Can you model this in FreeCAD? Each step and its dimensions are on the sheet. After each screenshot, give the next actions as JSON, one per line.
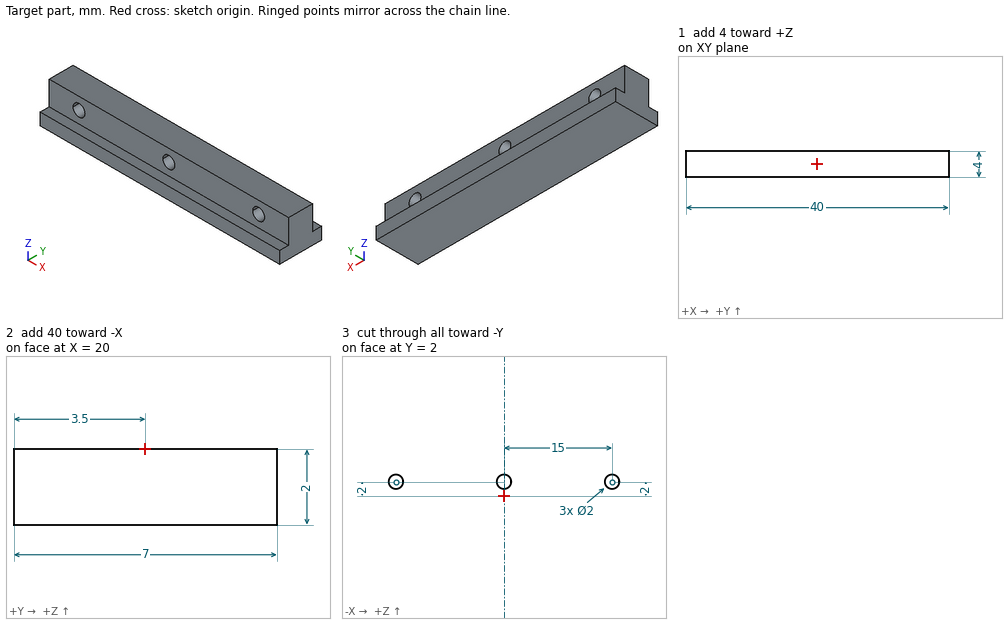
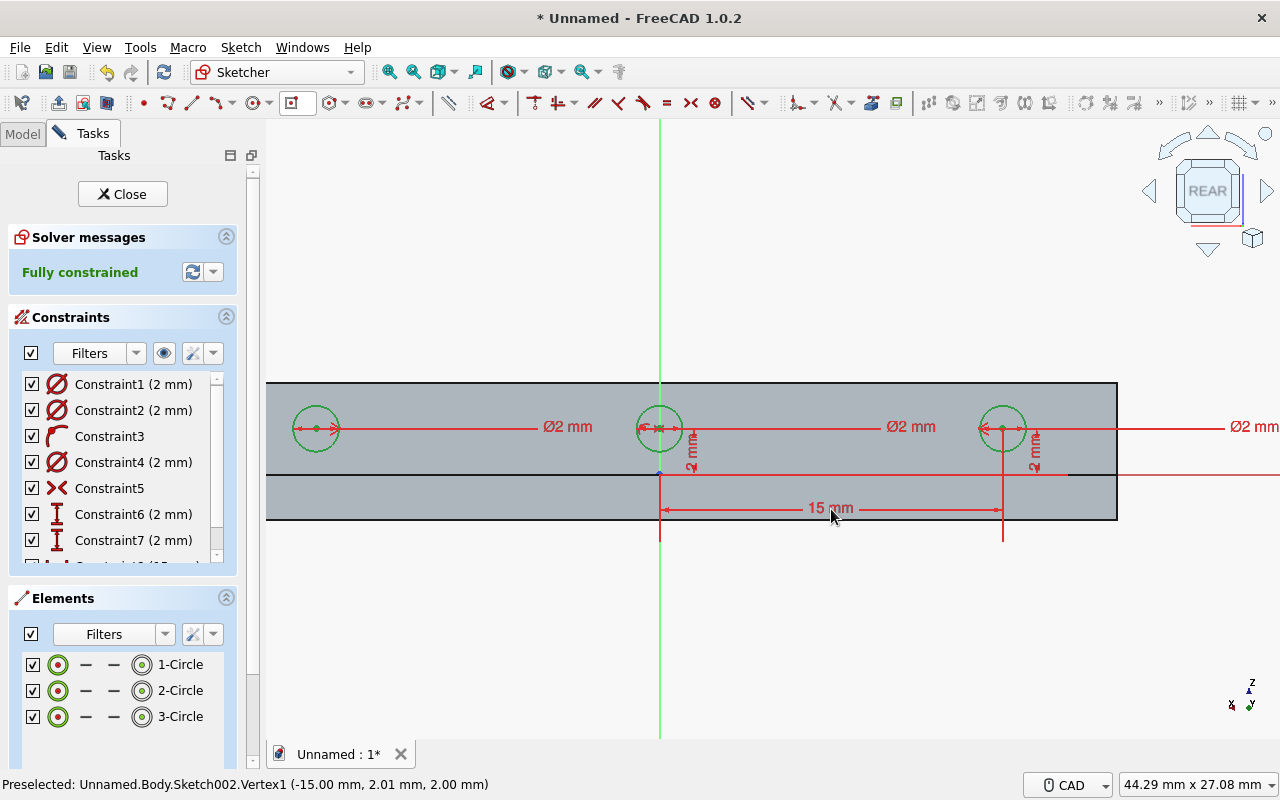
{"action": "left_click", "coordinate": [123, 194]}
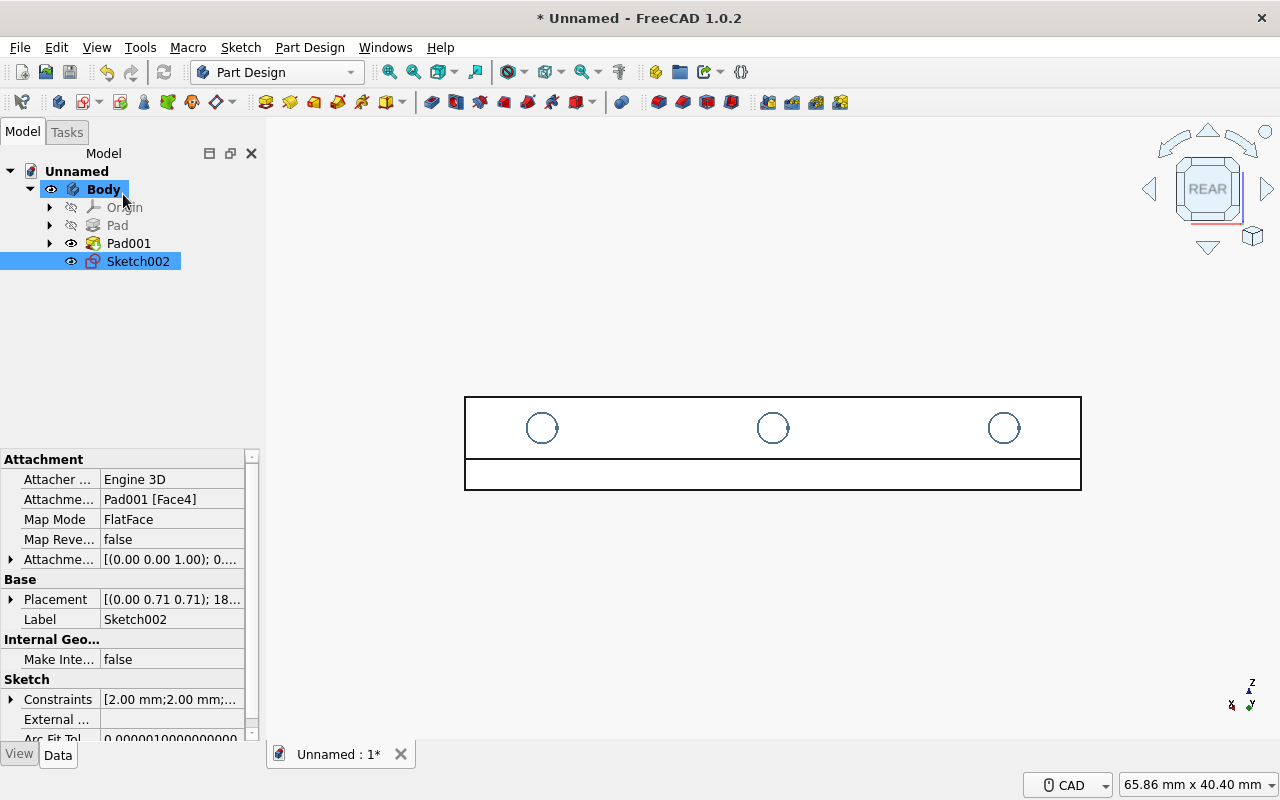
{"action": "left_click", "coordinate": [432, 102]}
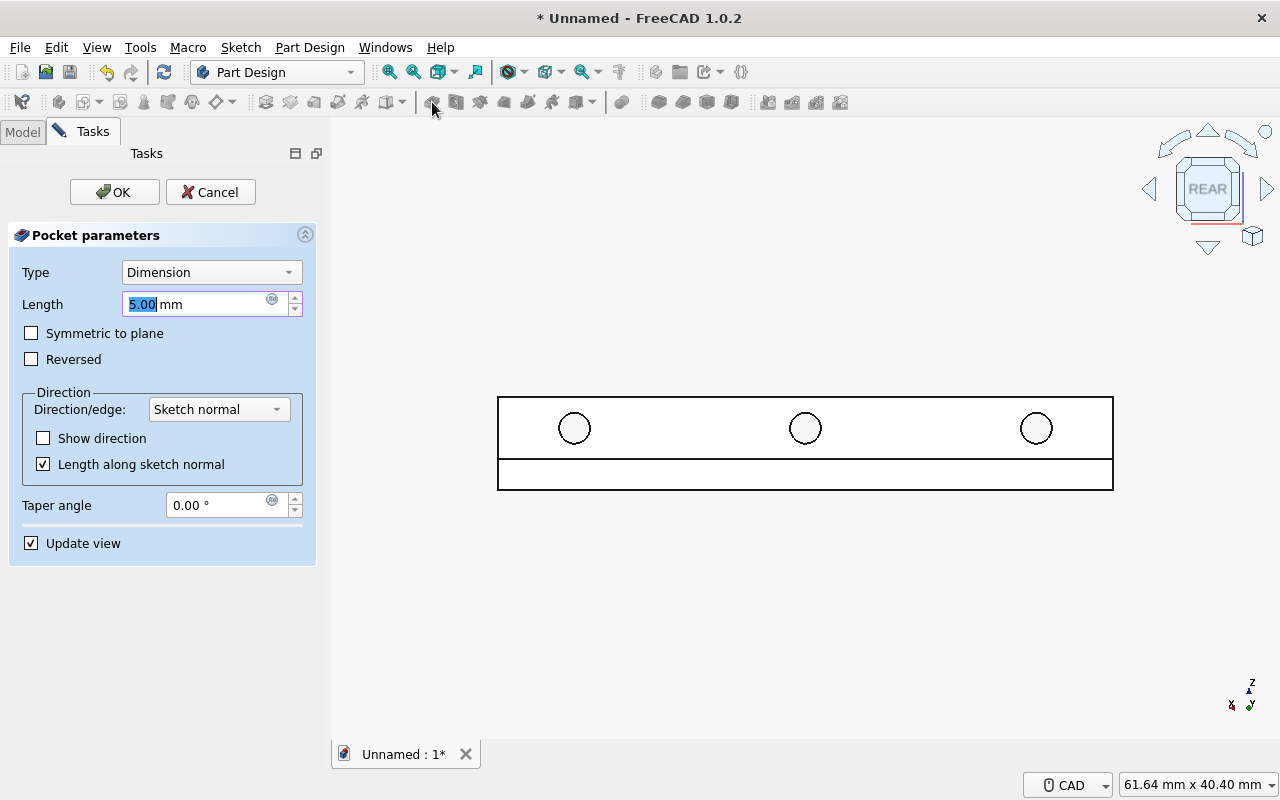
{"action": "left_click", "coordinate": [212, 272]}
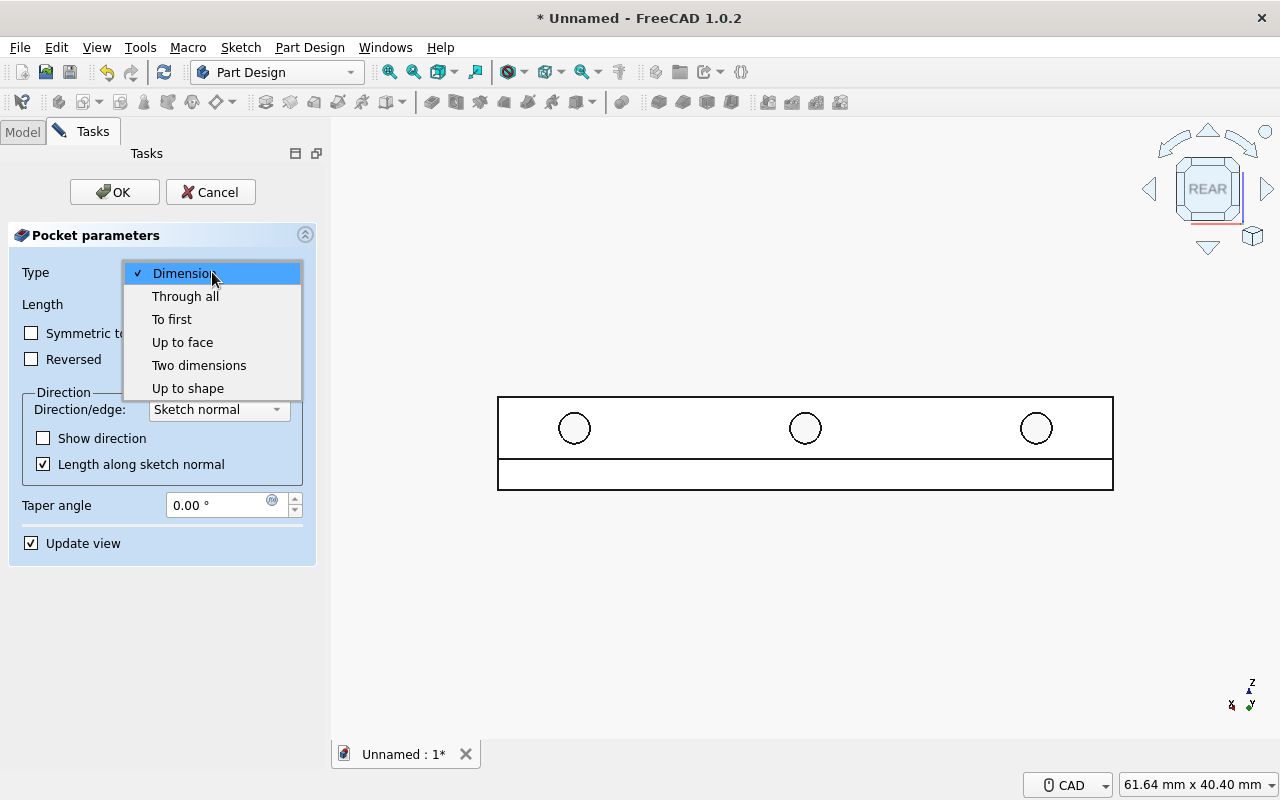
{"action": "left_click", "coordinate": [212, 296]}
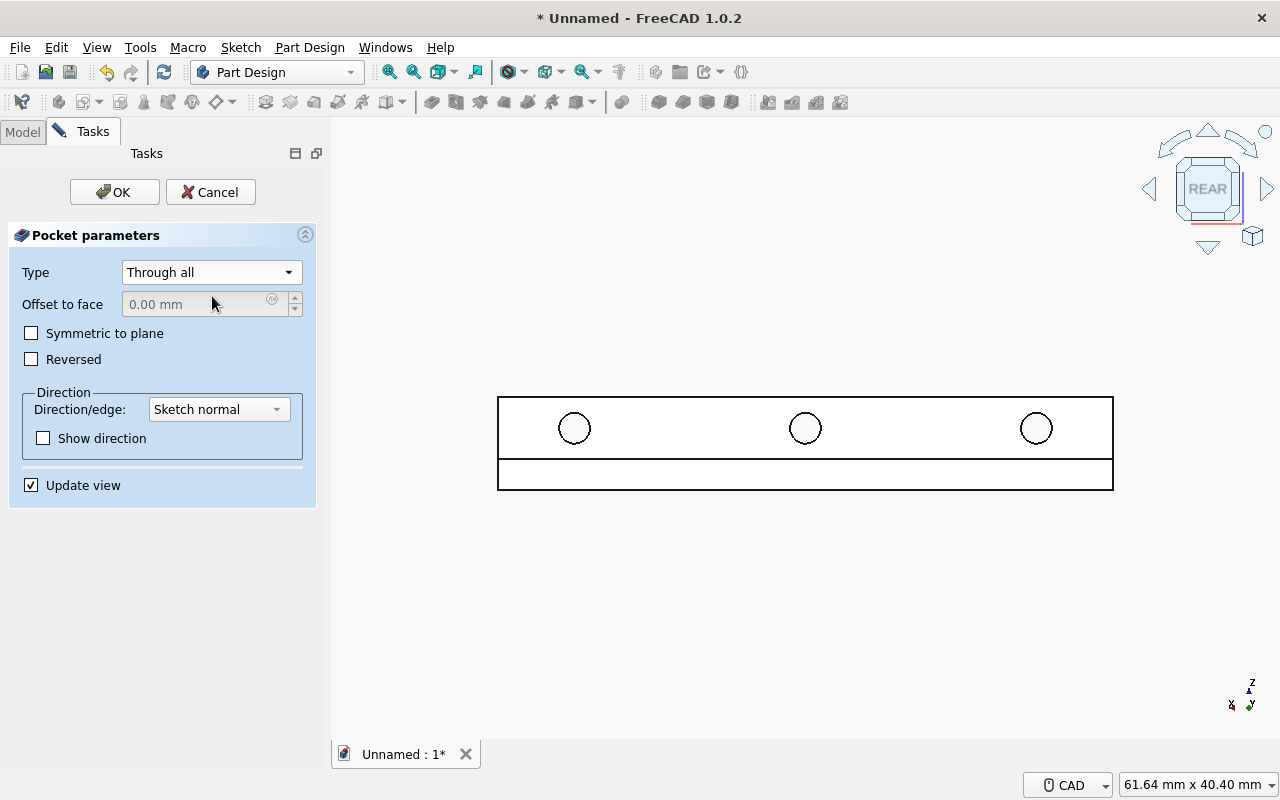
{"action": "left_click", "coordinate": [115, 192]}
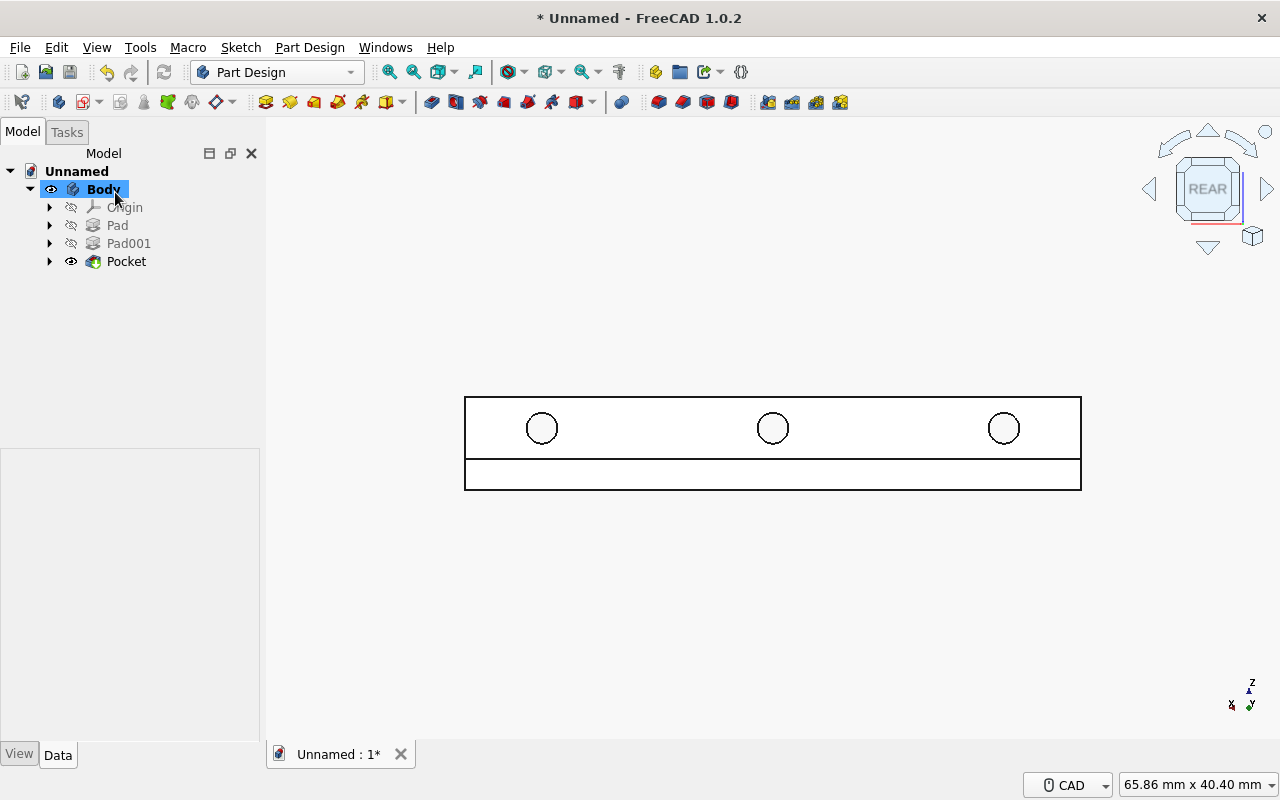
{"action": "key", "text": "0"}